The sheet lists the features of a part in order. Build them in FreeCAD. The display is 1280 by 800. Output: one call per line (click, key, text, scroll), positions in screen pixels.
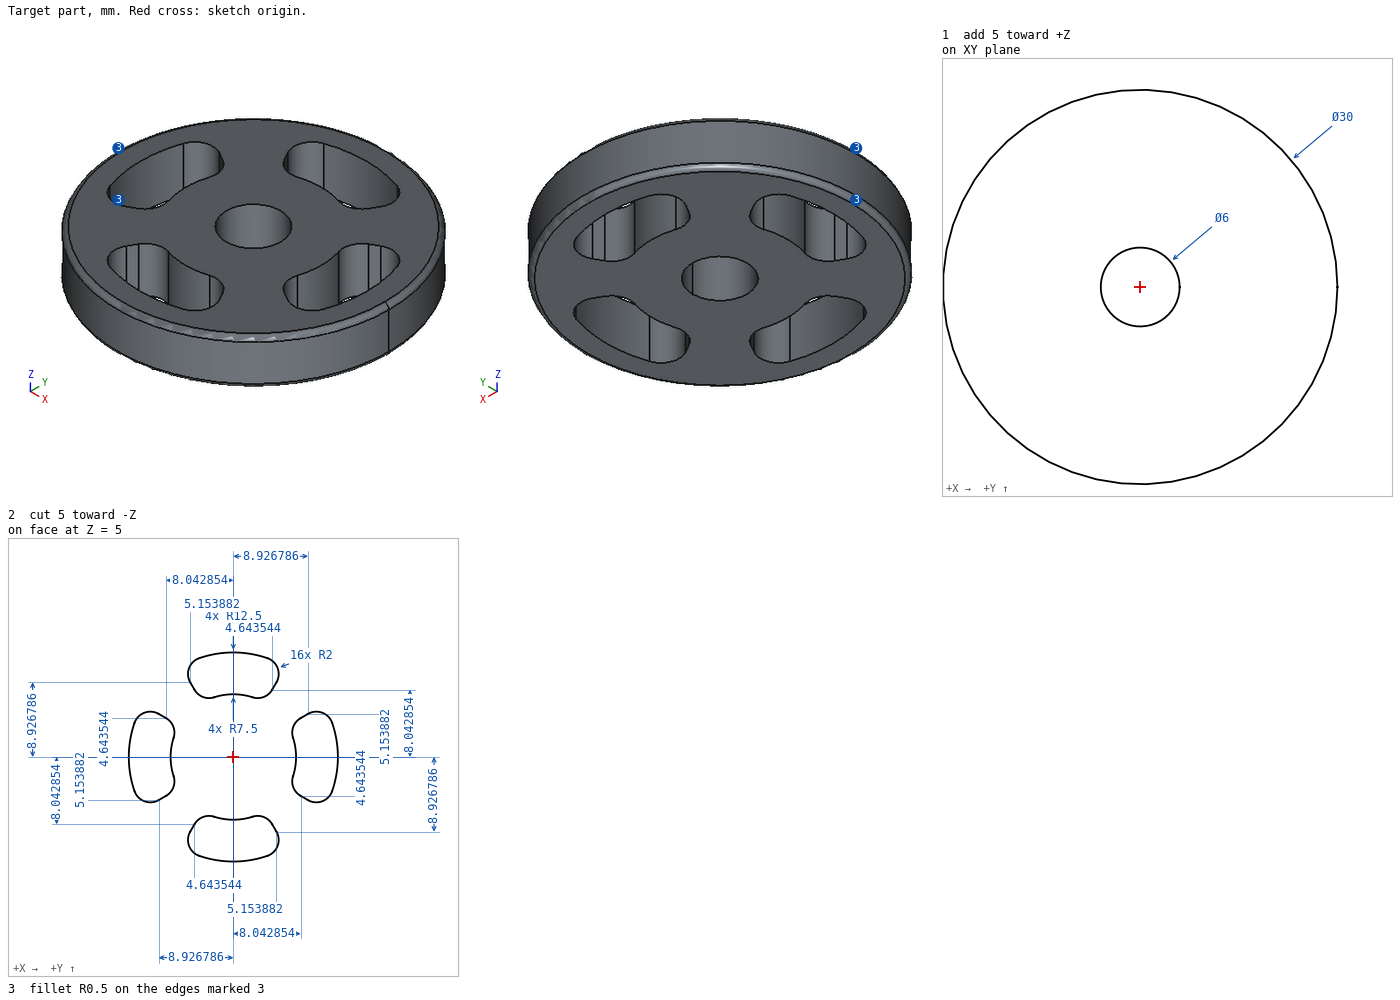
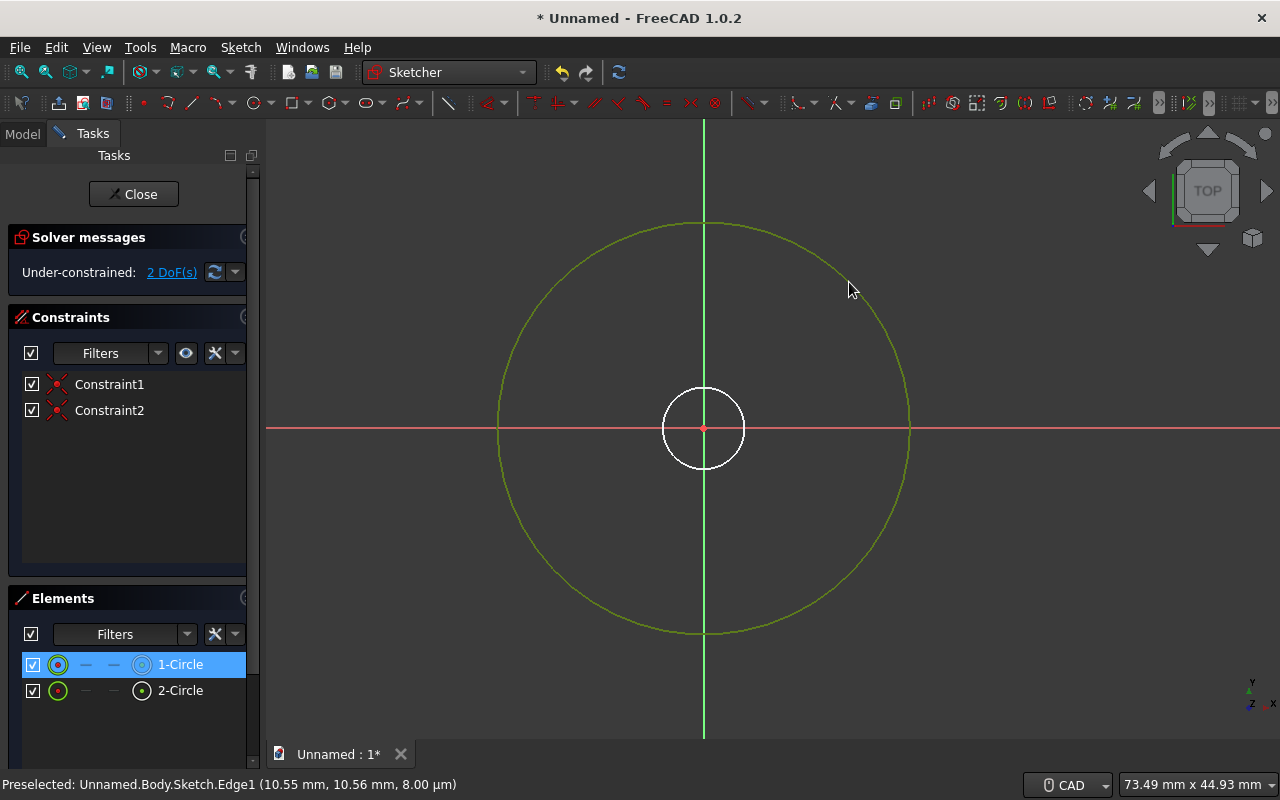
key(k)
key(o)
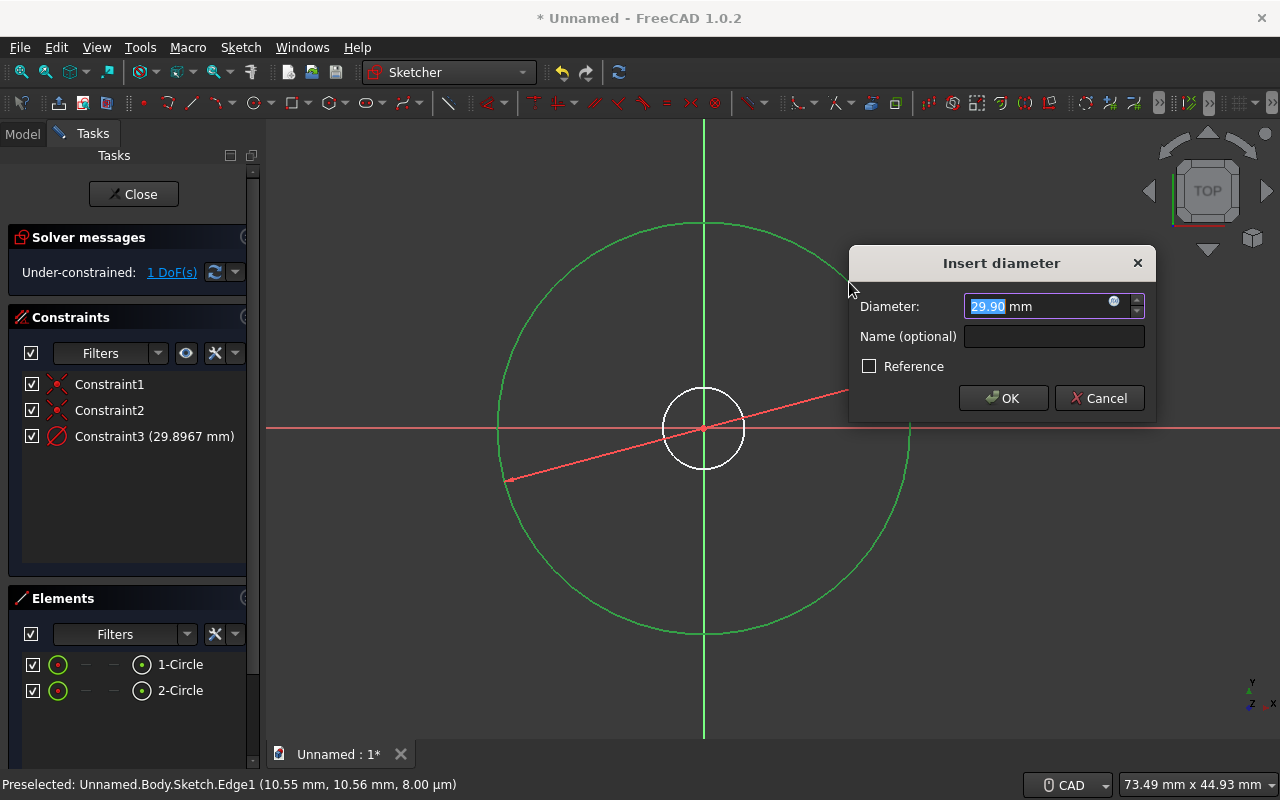
text(30)
key(Return)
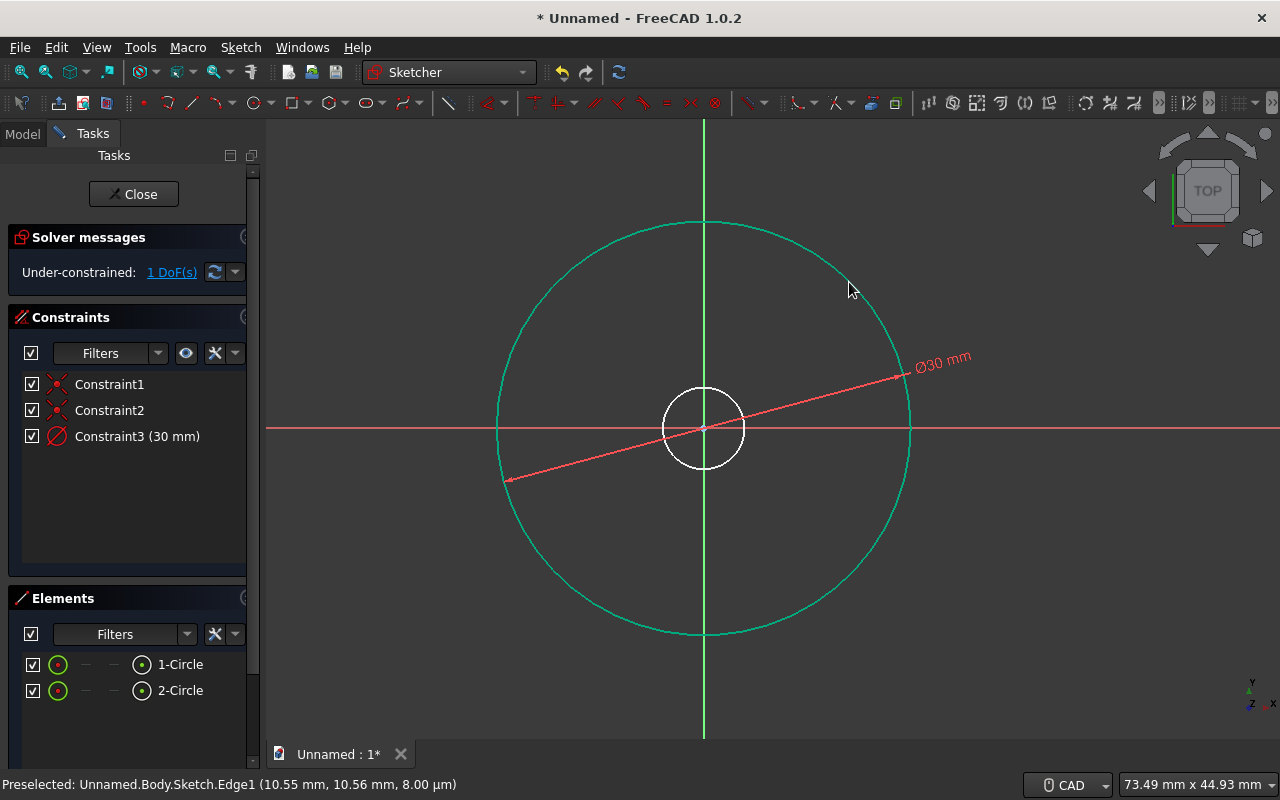
click(732, 399)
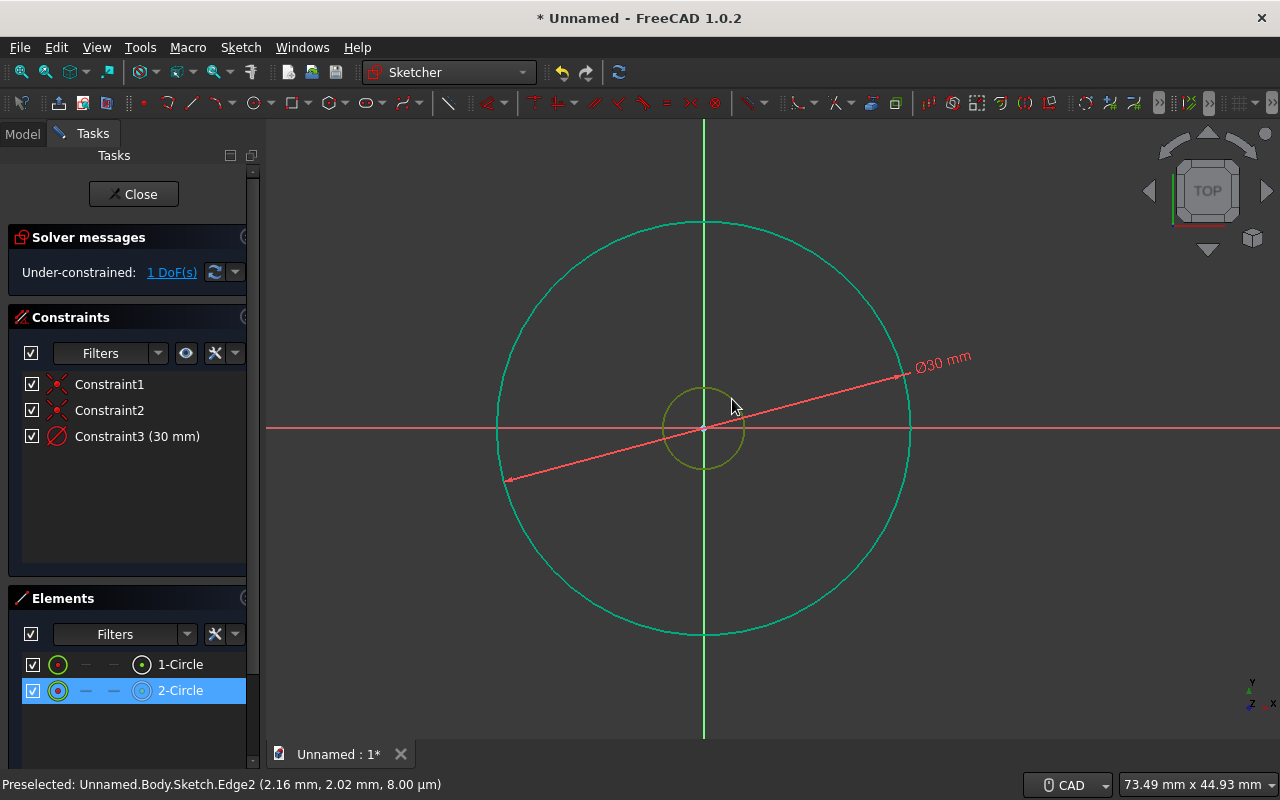
click(506, 104)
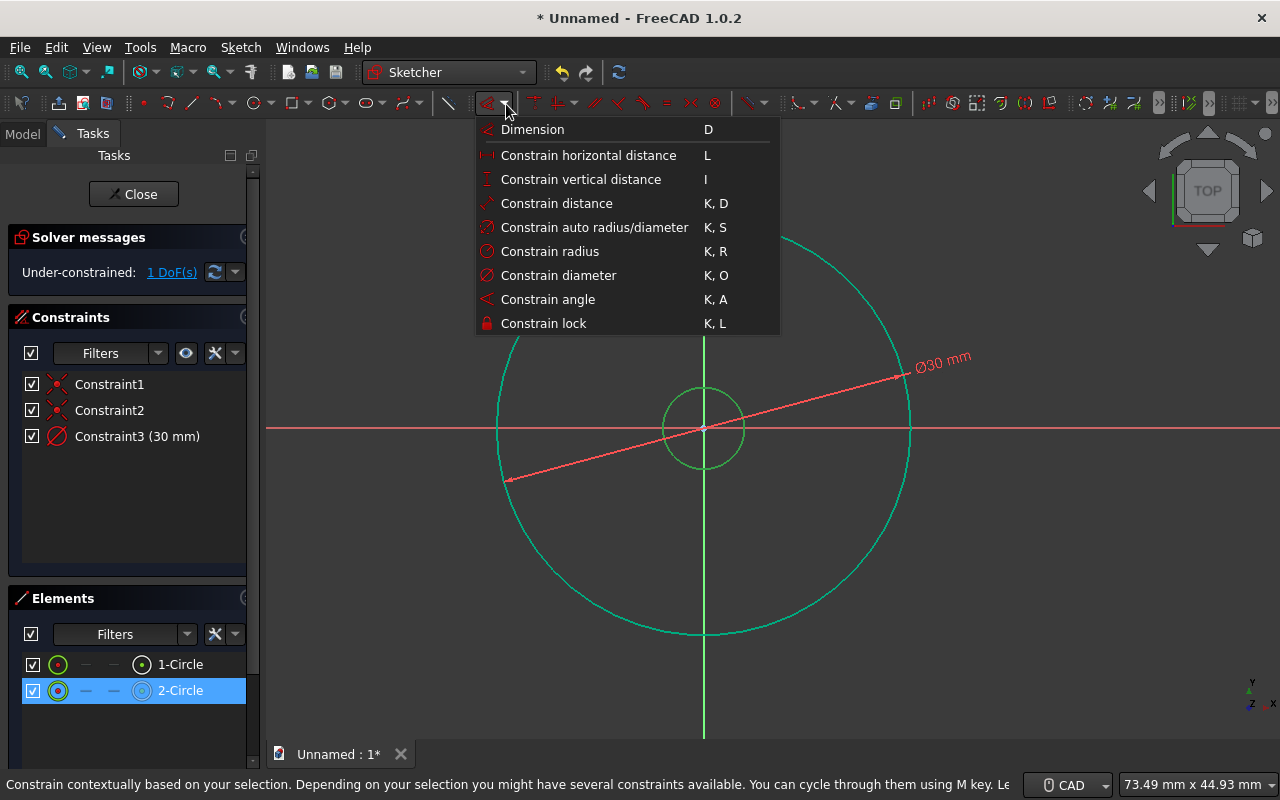
click(628, 275)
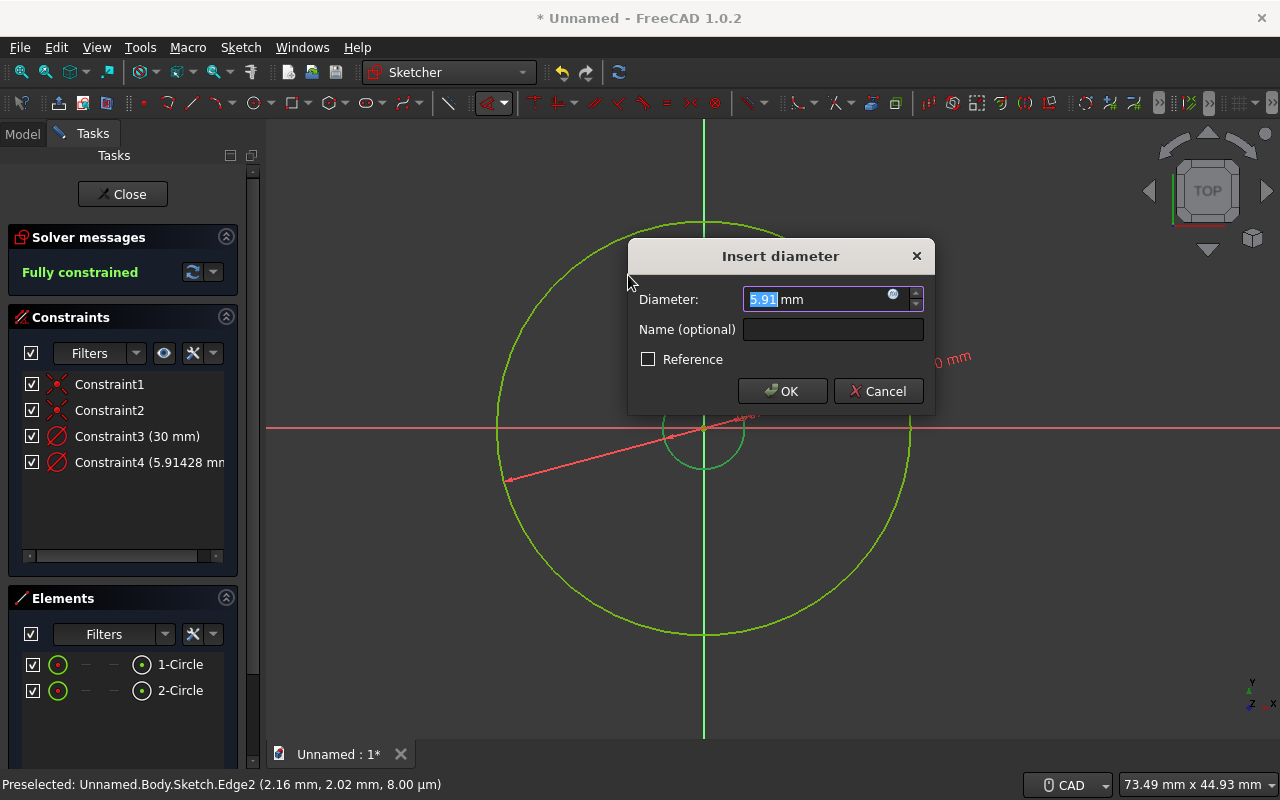
text(6)
key(Return)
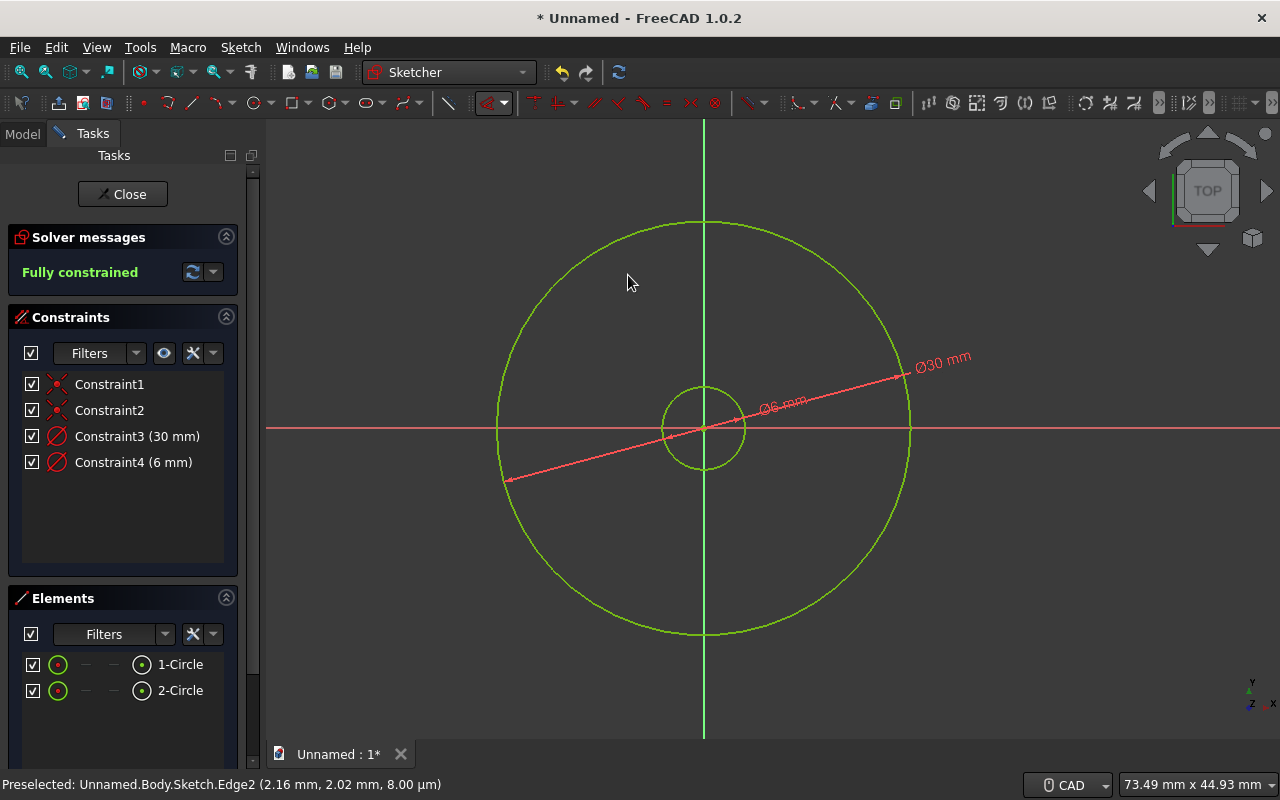
click(123, 194)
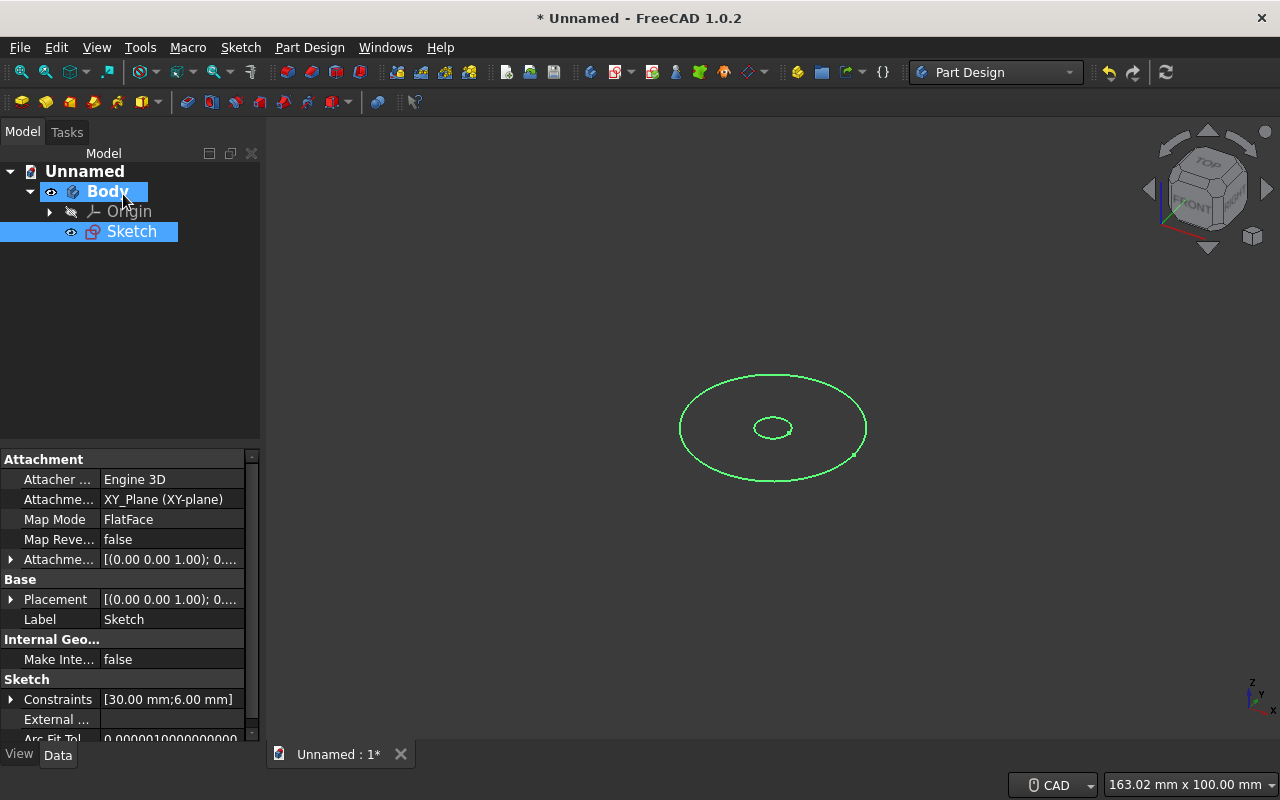
click(22, 102)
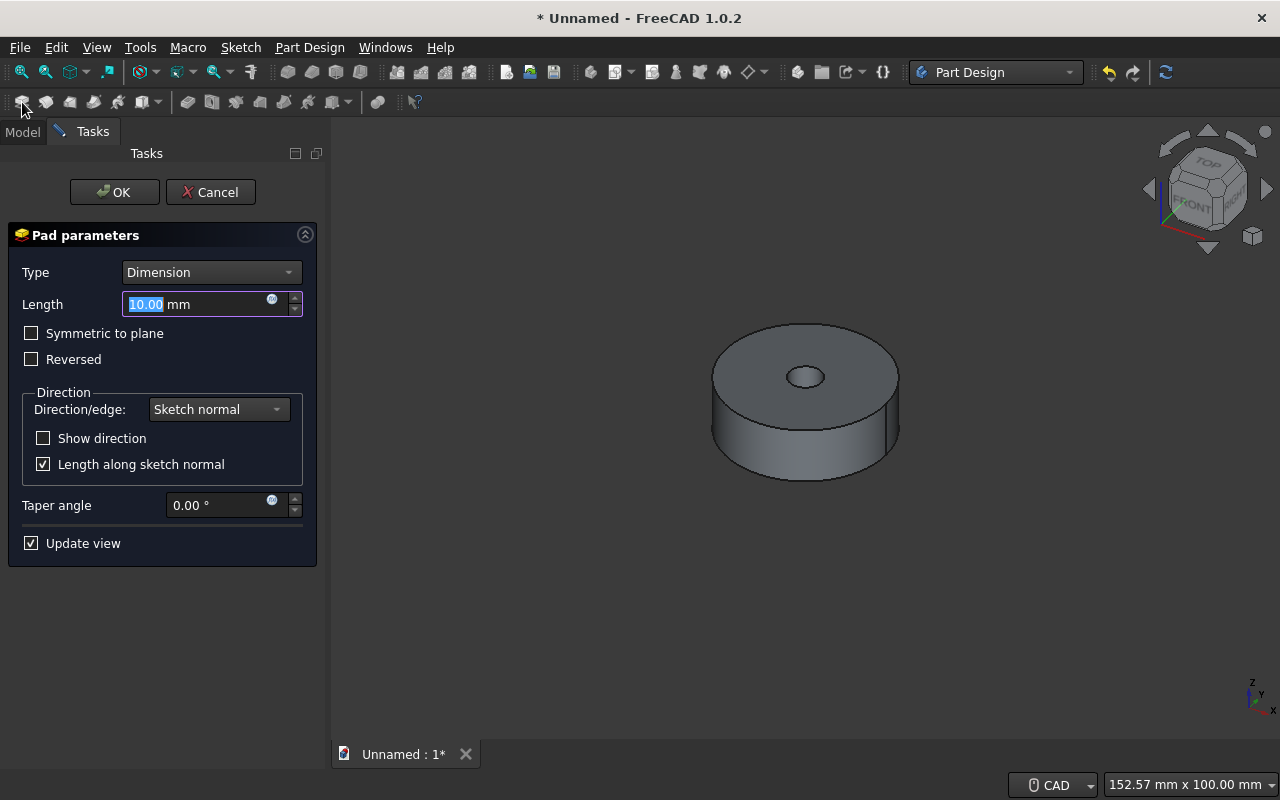
text(5)
key(Tab)